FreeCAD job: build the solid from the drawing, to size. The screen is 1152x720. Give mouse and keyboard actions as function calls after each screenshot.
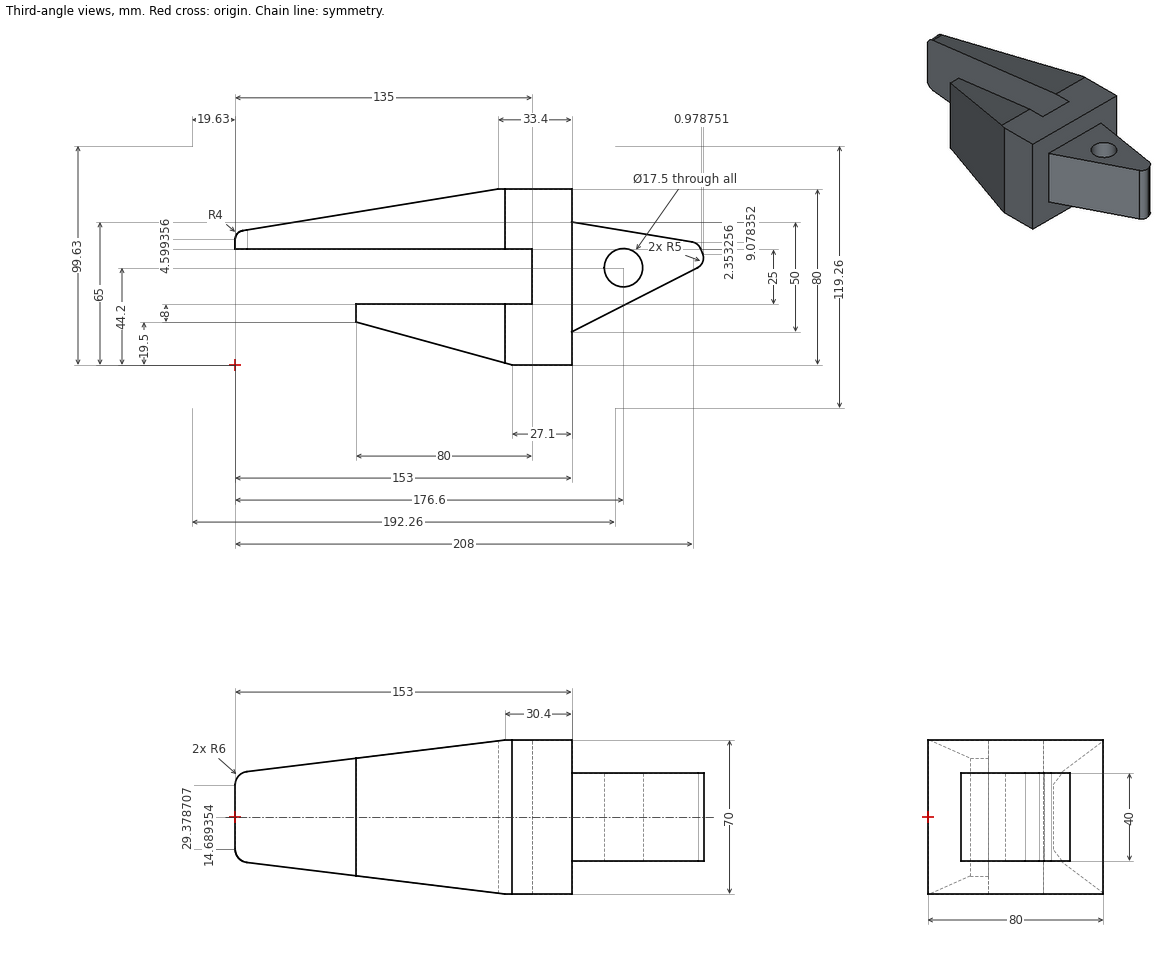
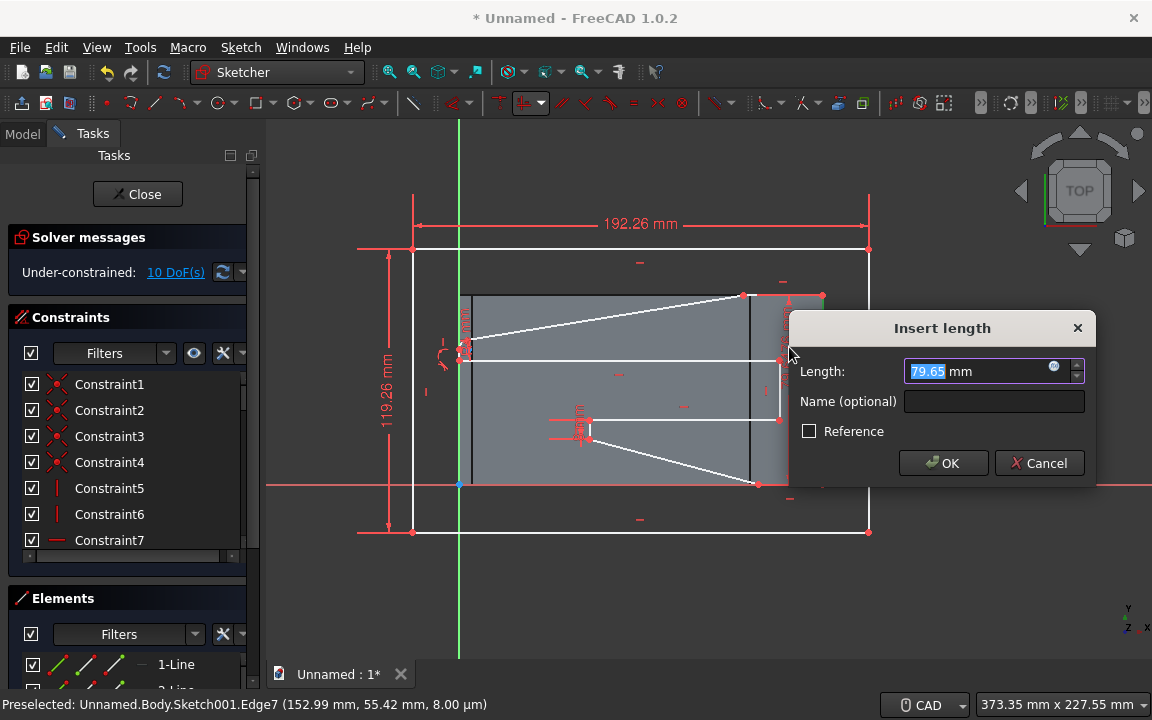
text(80)
key(Return)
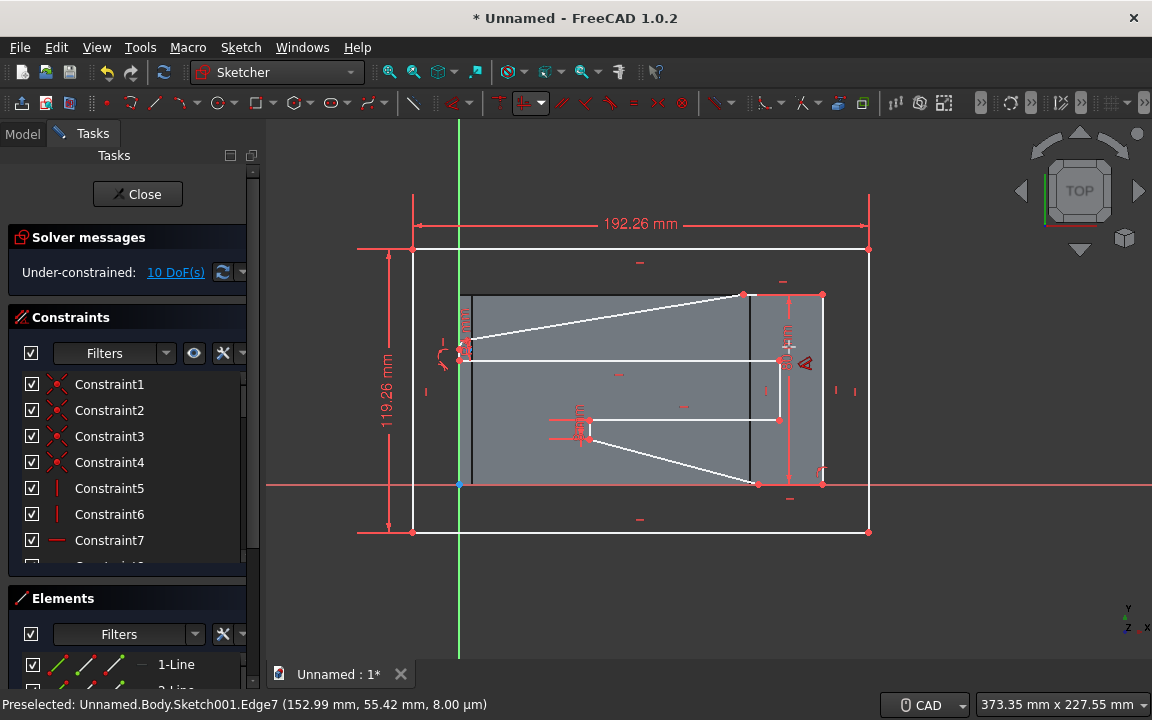
click(647, 420)
click(728, 454)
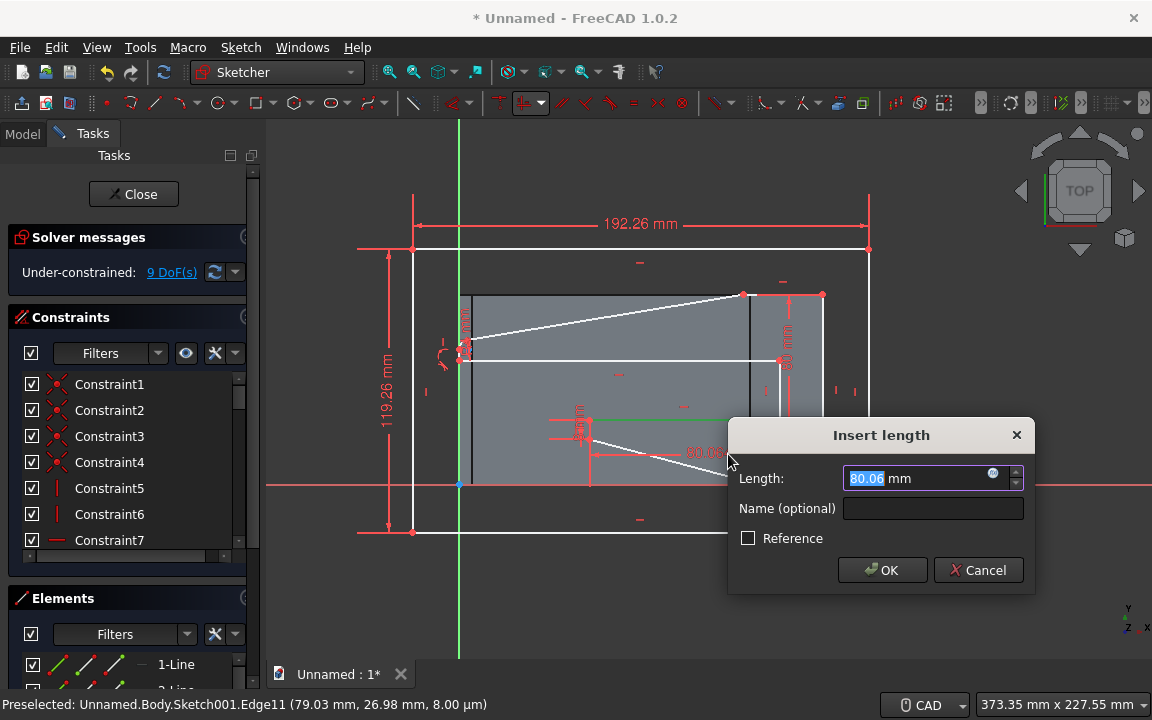
text(80)
key(Return)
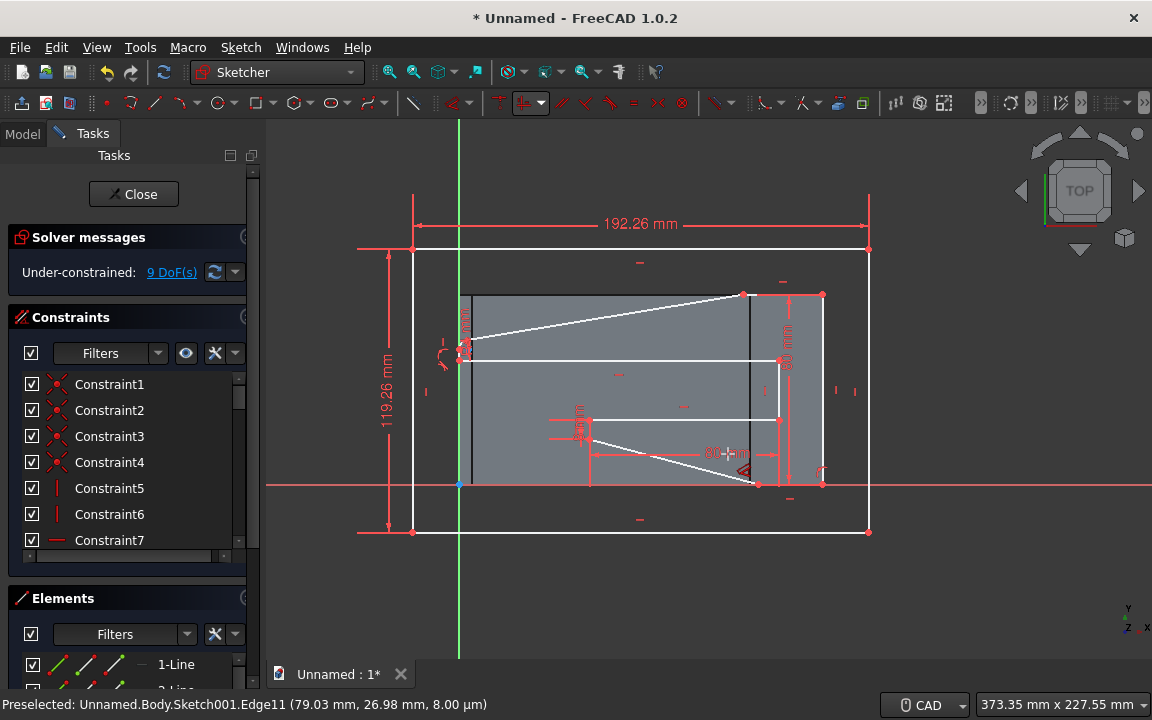
click(779, 403)
click(745, 391)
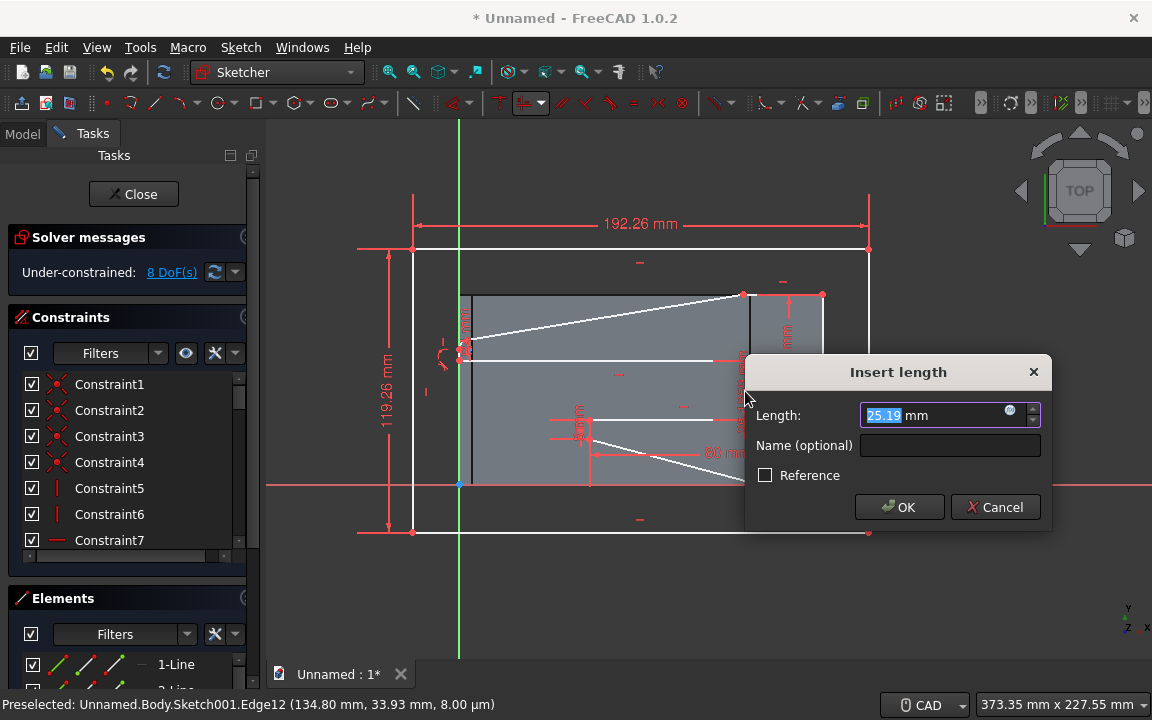
text(25)
key(Return)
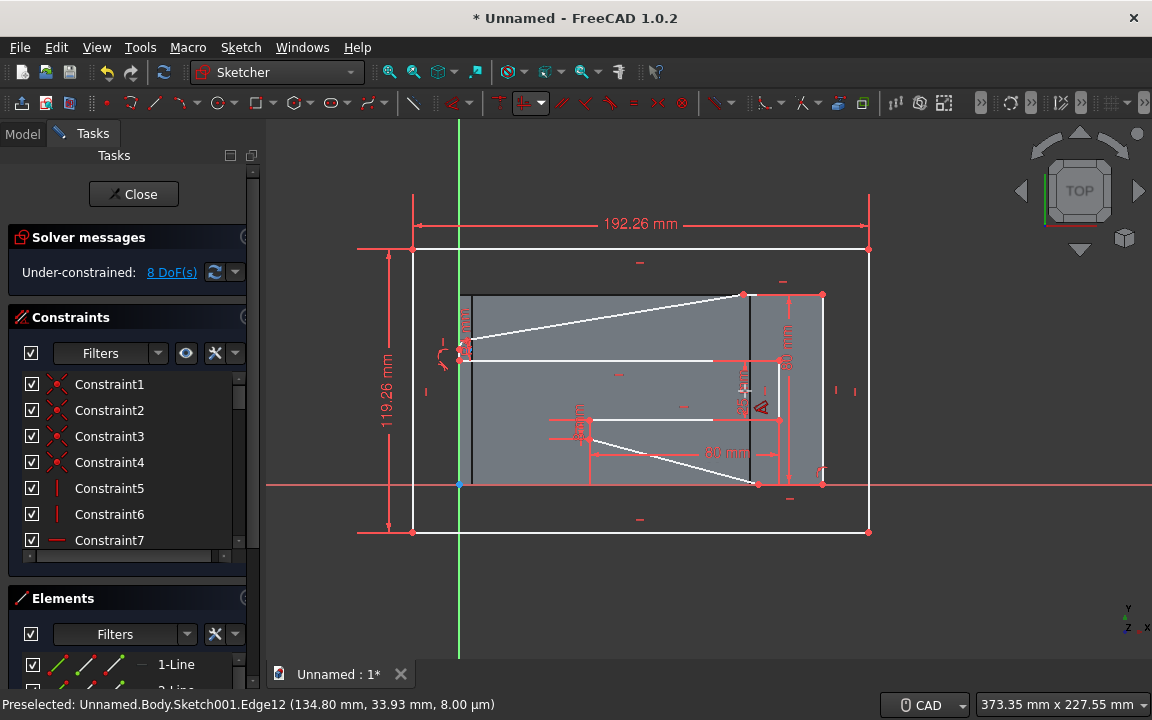
click(683, 361)
click(693, 327)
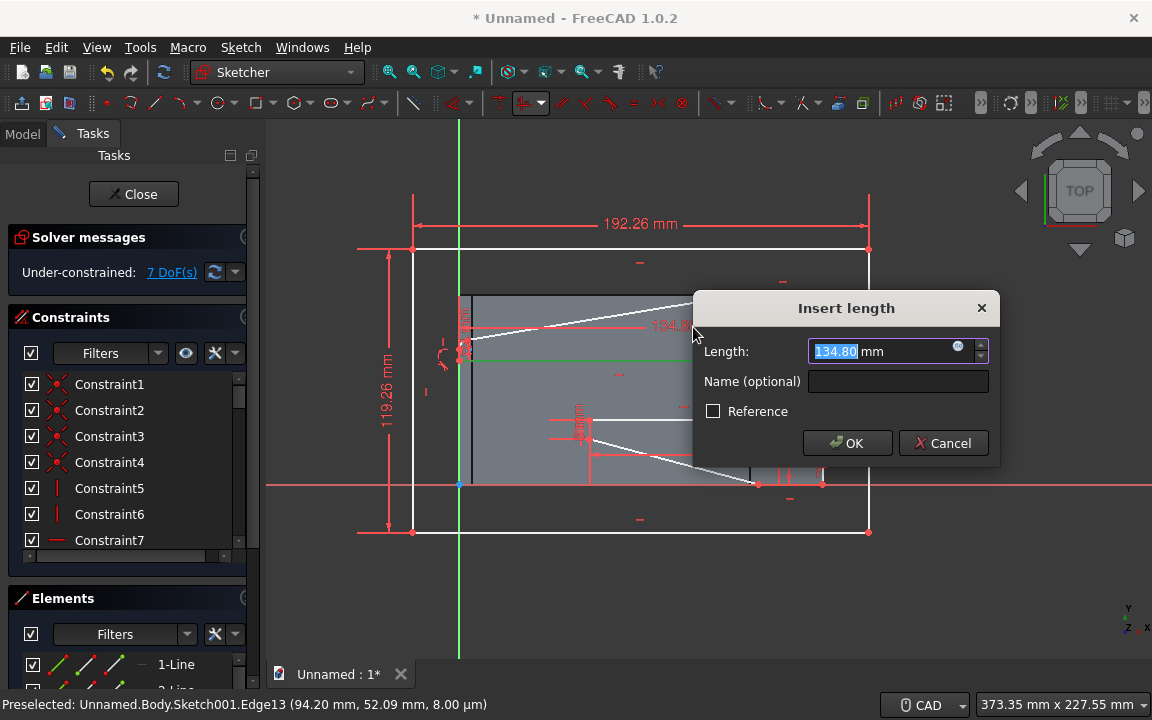
text(135)
key(Return)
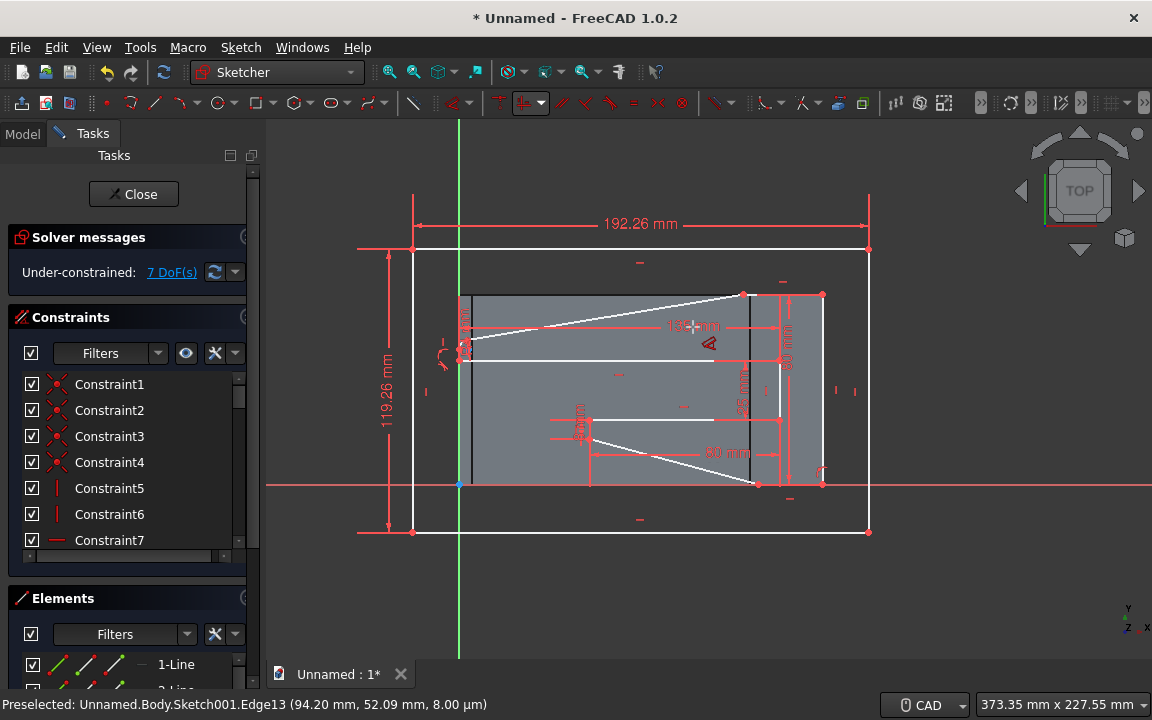
click(767, 295)
click(783, 213)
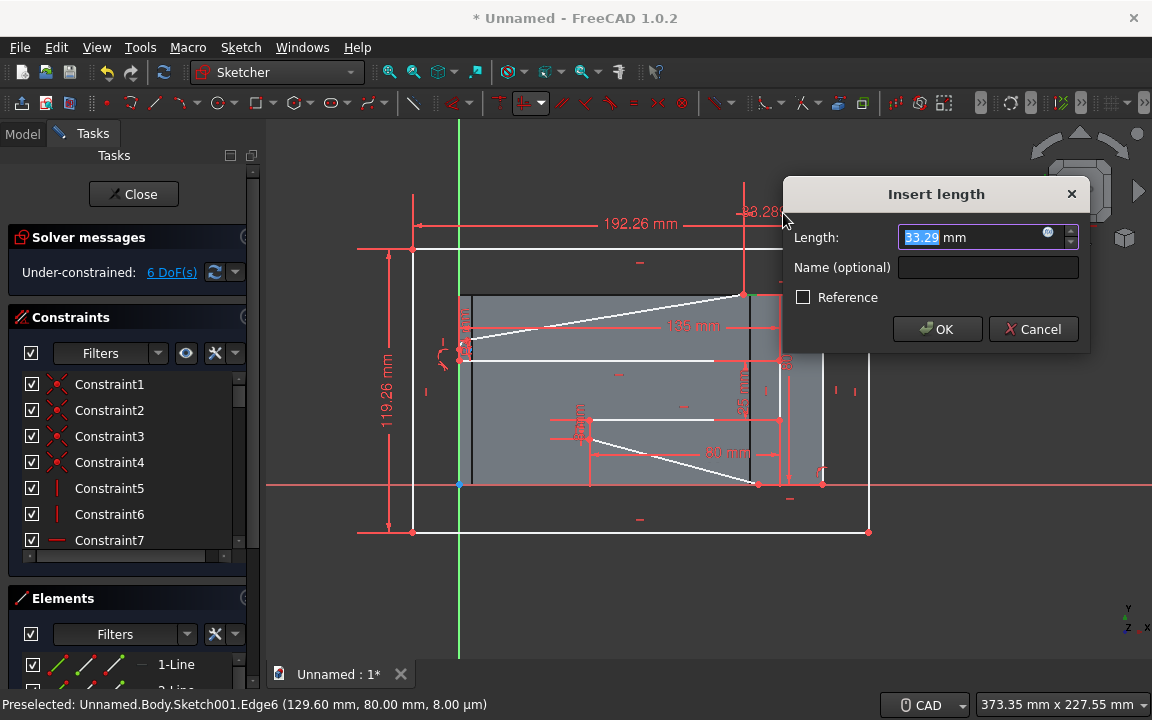
text(33.4)
key(Return)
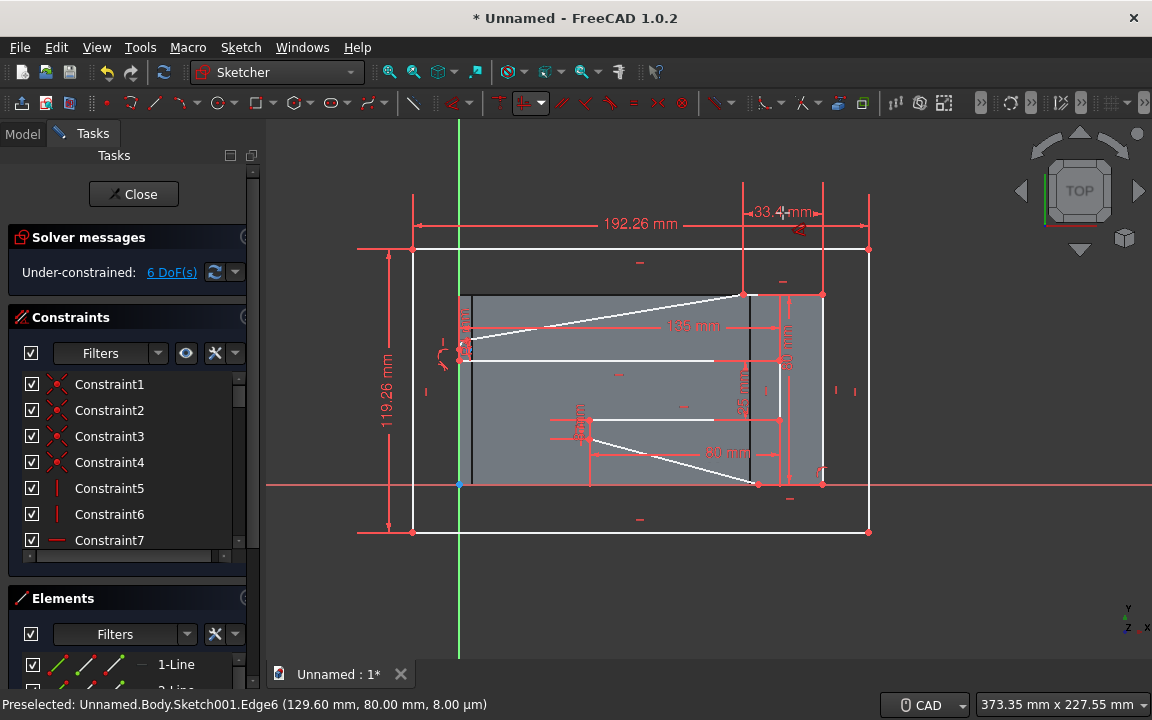
click(803, 485)
click(791, 519)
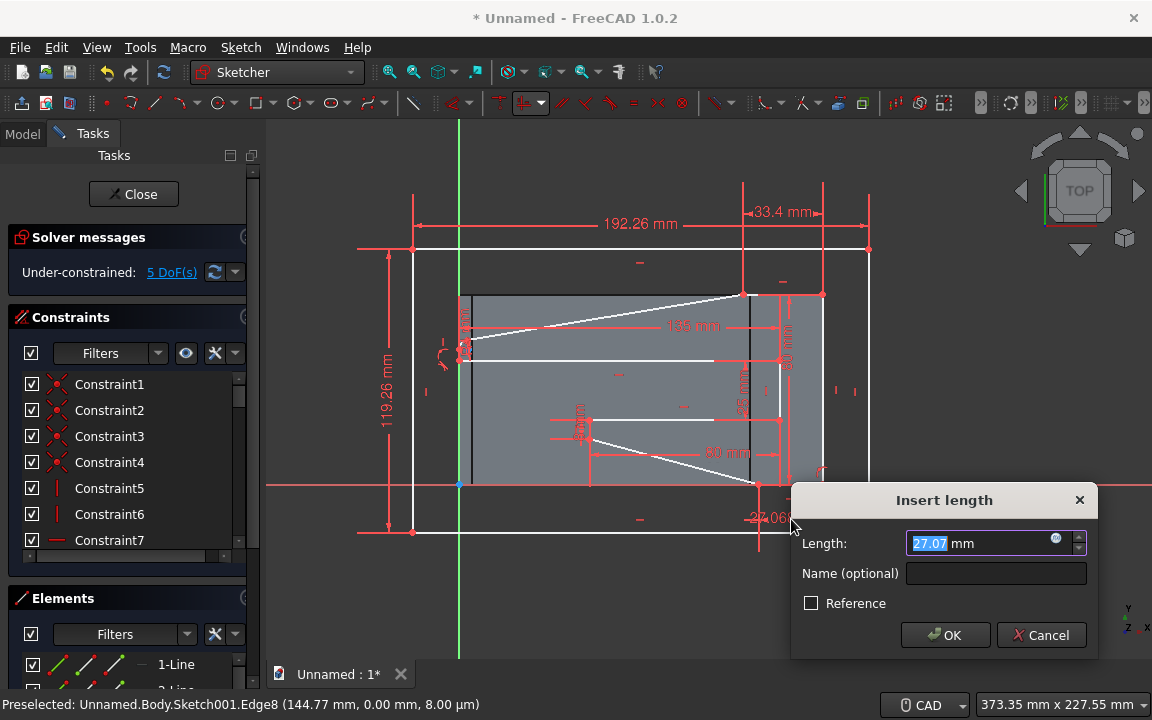
text(27.1)
key(Return)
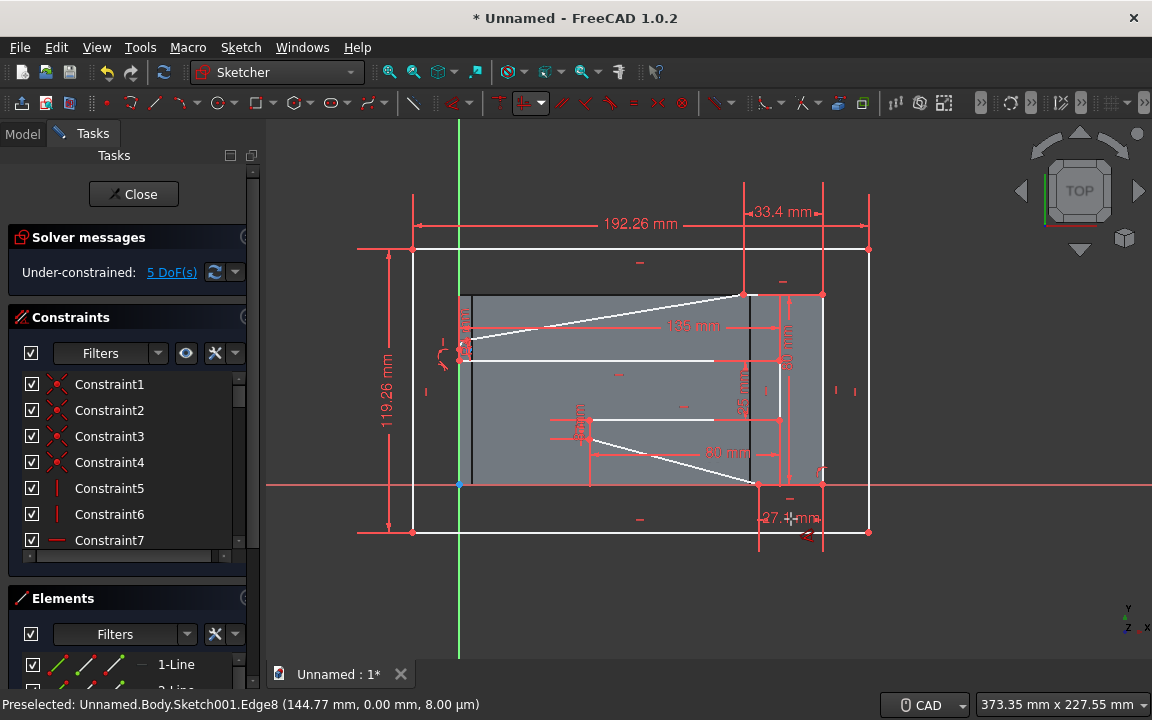
click(823, 295)
click(641, 519)